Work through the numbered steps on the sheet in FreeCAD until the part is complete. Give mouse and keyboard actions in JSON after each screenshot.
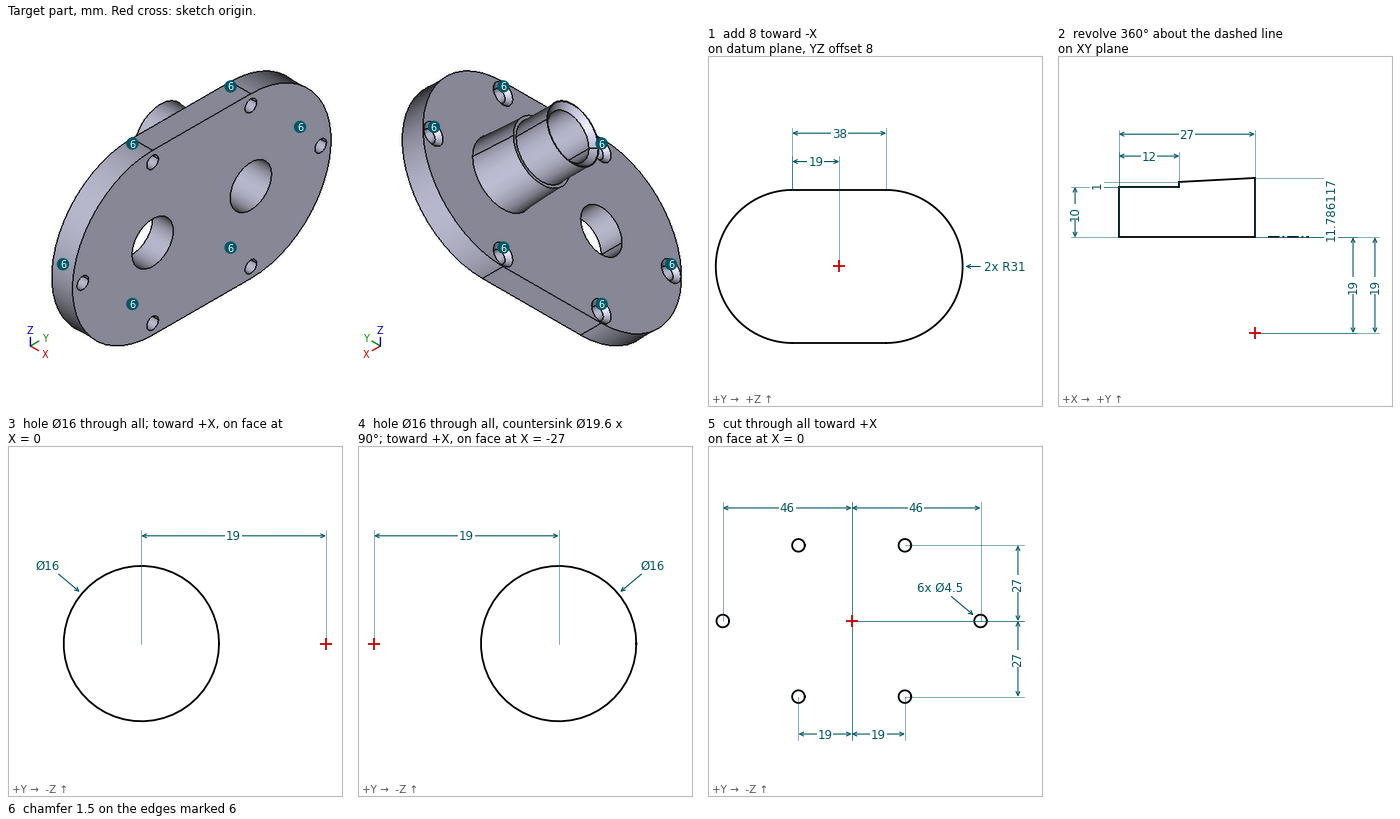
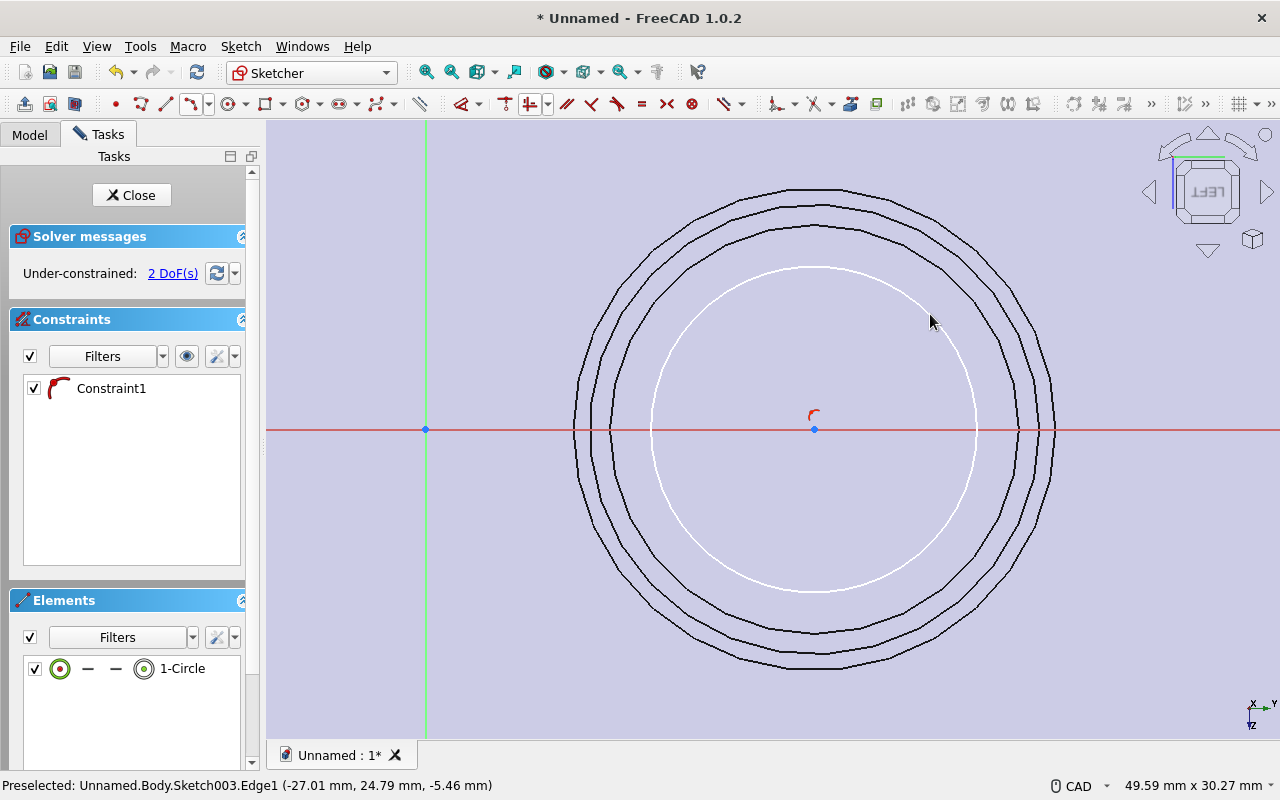
{"action": "key", "text": "d"}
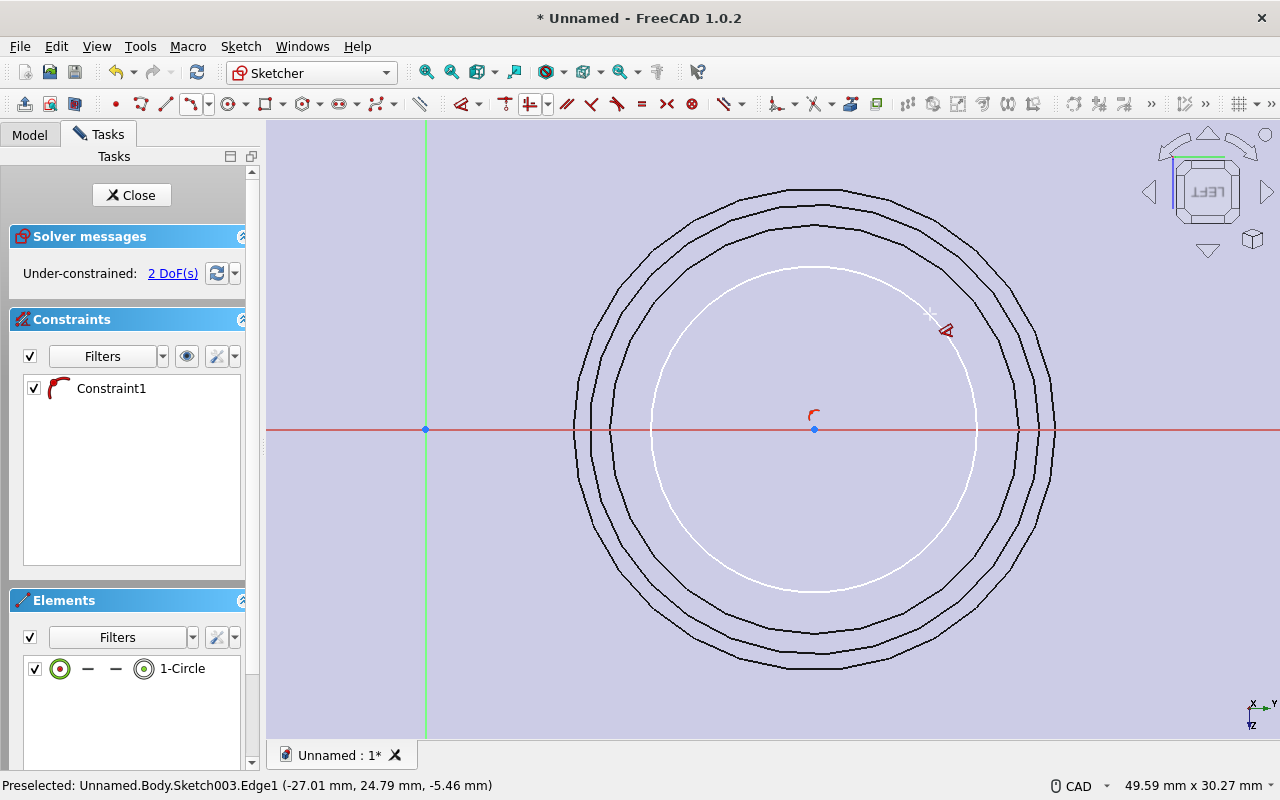
{"action": "left_click", "coordinate": [929, 314]}
{"action": "left_click", "coordinate": [952, 291]}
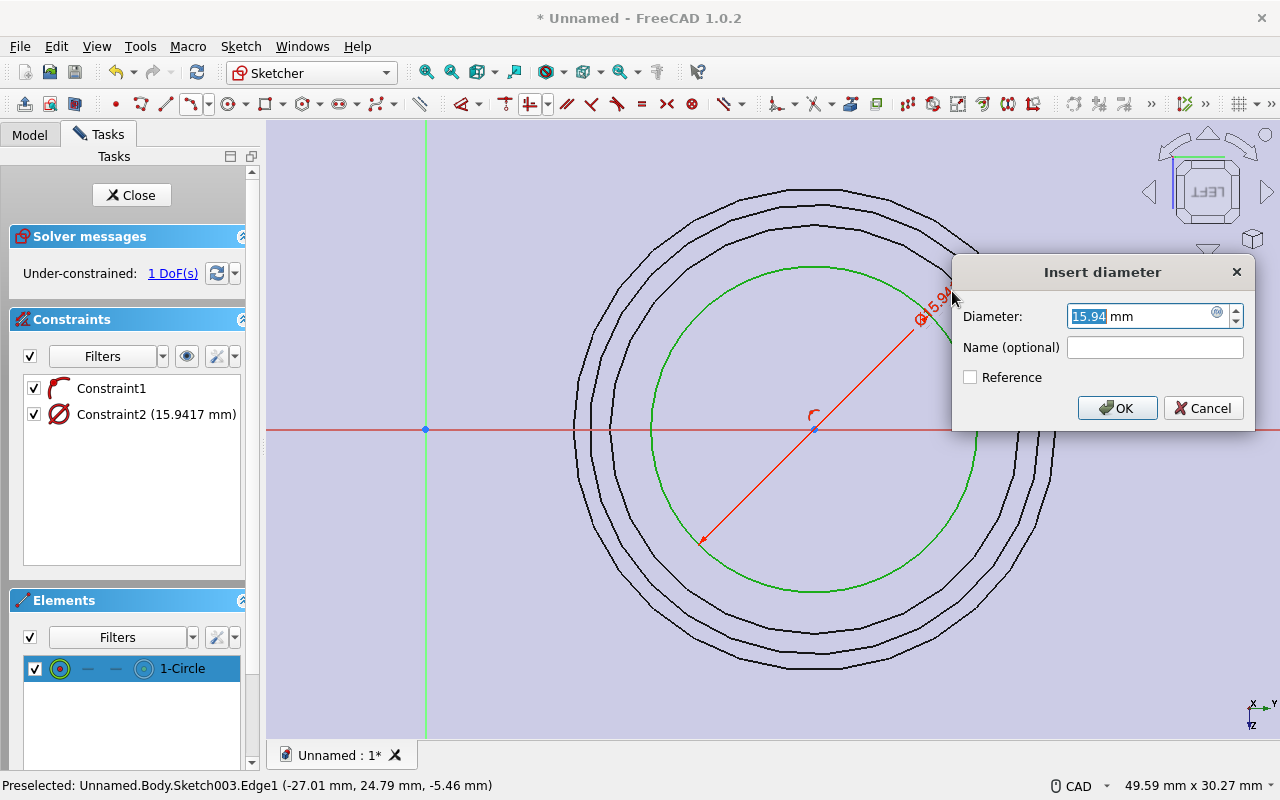
{"action": "type", "text": "16"}
{"action": "key", "text": "Return"}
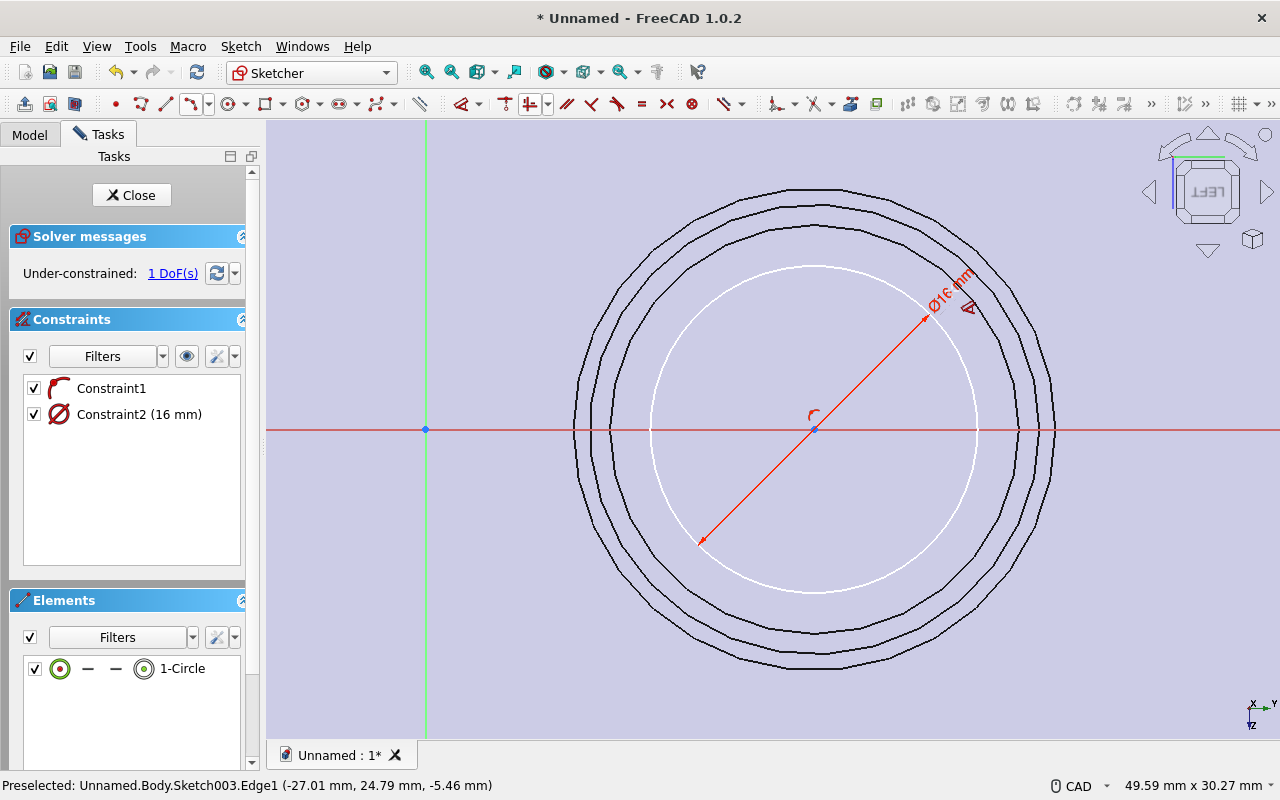
{"action": "left_click", "coordinate": [814, 429]}
{"action": "left_click", "coordinate": [620, 463]}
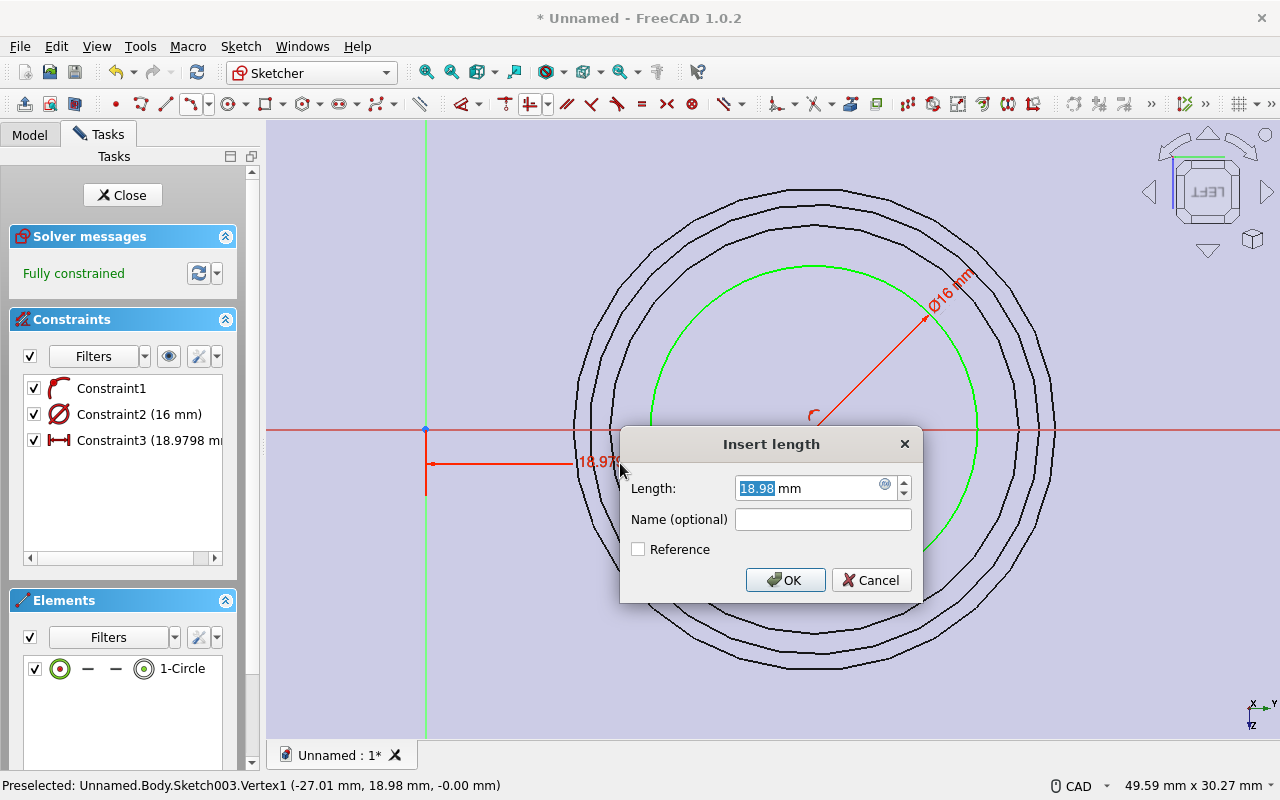
{"action": "type", "text": "19"}
{"action": "key", "text": "Return"}
{"action": "key", "text": "Escape"}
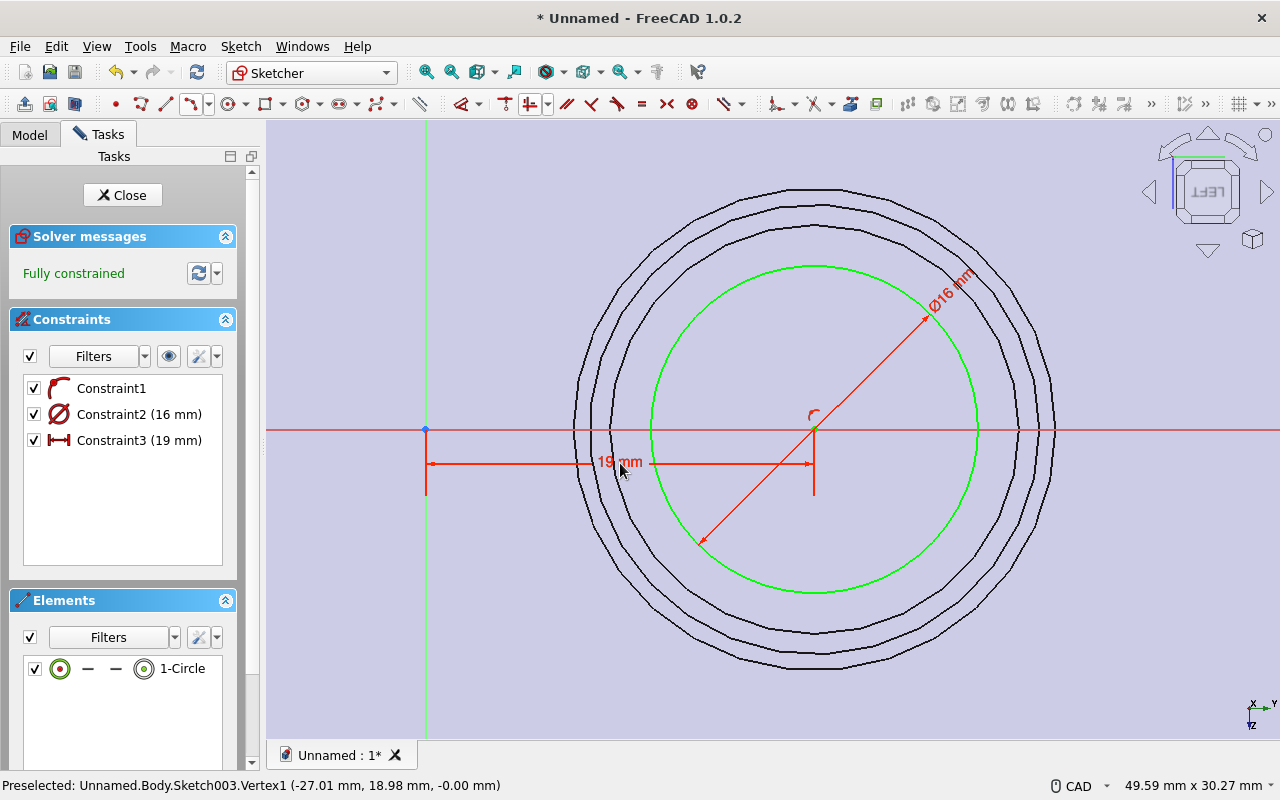
{"action": "left_click", "coordinate": [123, 195]}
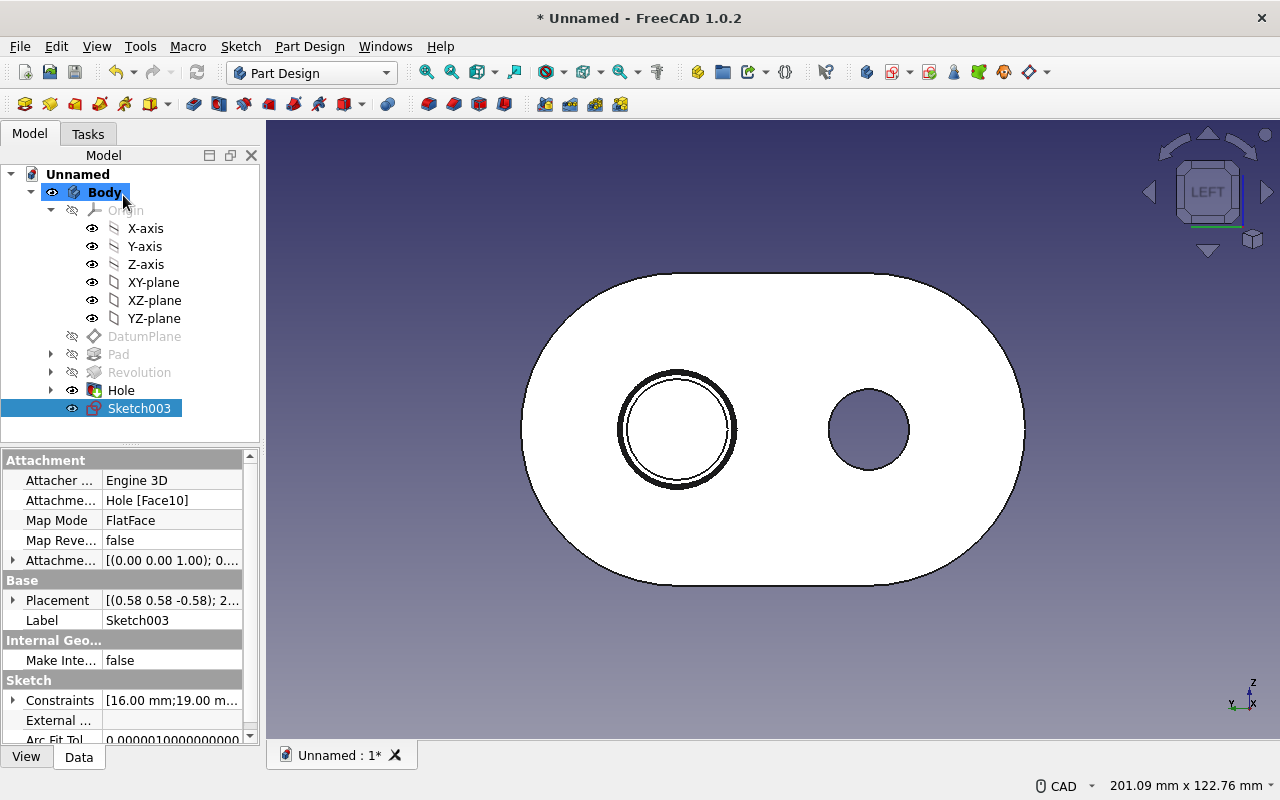
{"action": "left_click", "coordinate": [219, 104]}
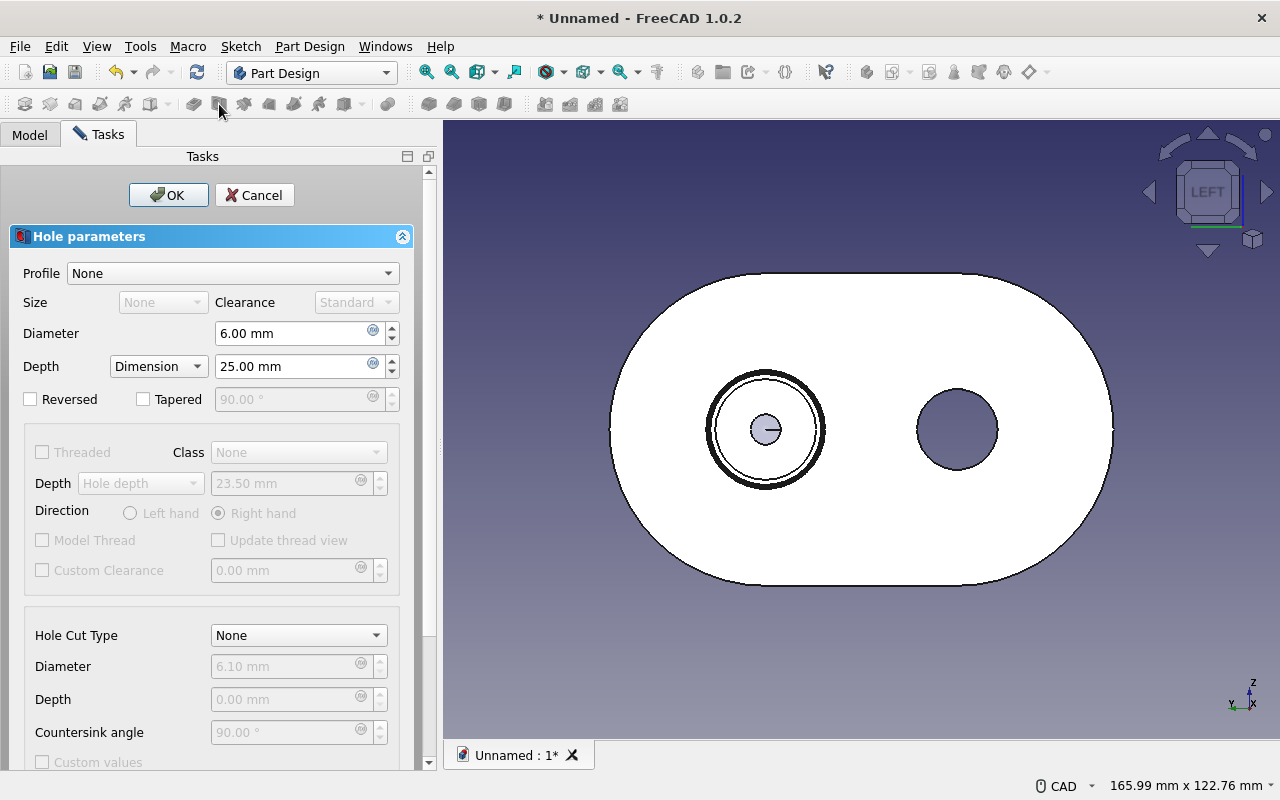
{"action": "triple_click", "coordinate": [300, 334]}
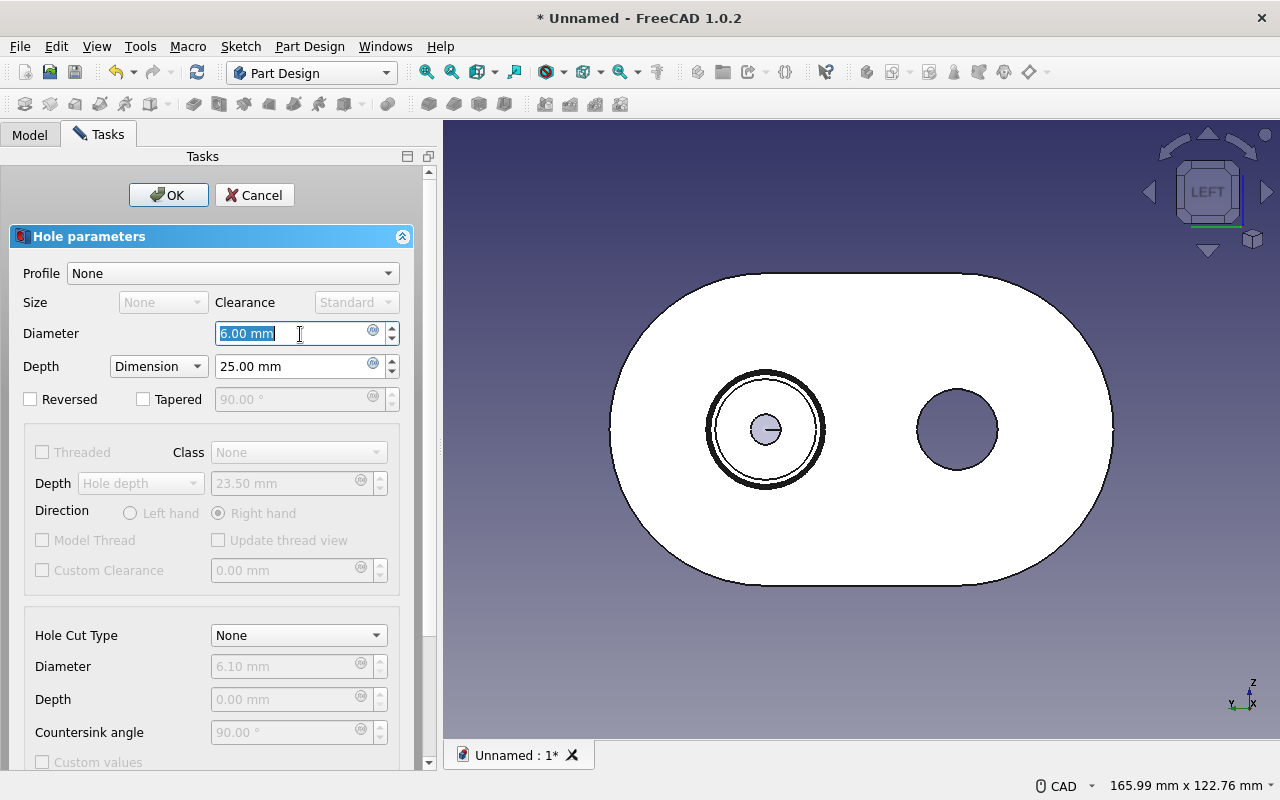
{"action": "type", "text": "16"}
{"action": "key", "text": "Tab"}